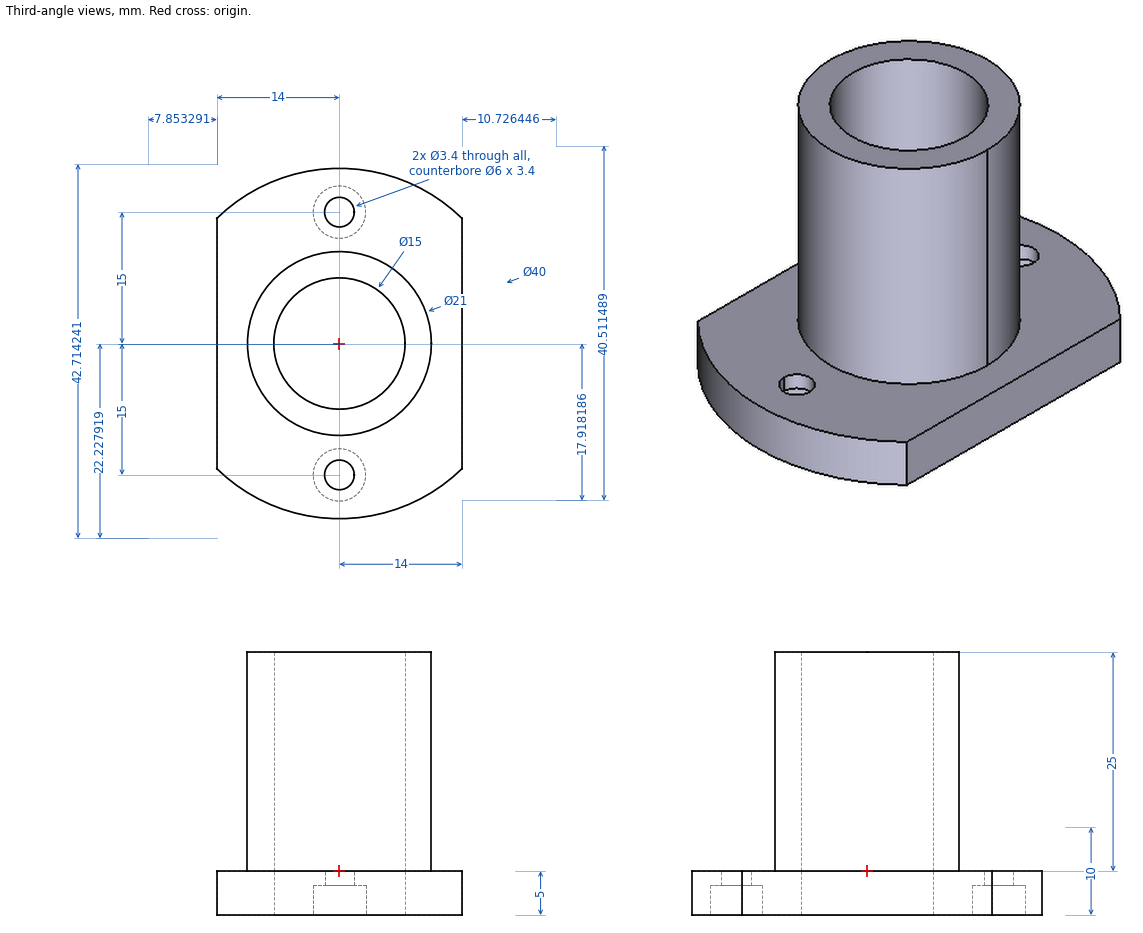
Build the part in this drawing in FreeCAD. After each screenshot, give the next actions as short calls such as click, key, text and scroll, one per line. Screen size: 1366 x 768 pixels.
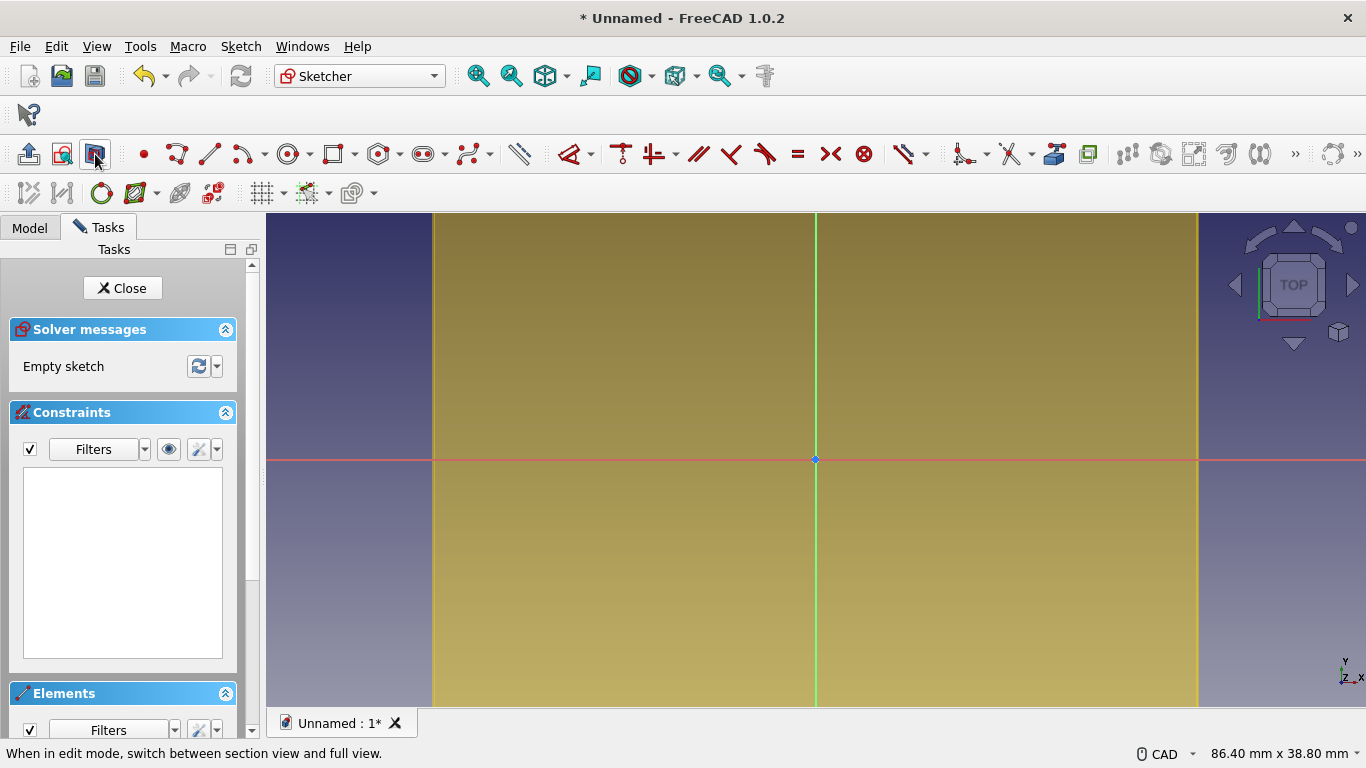
scroll(609, 460, down, 2)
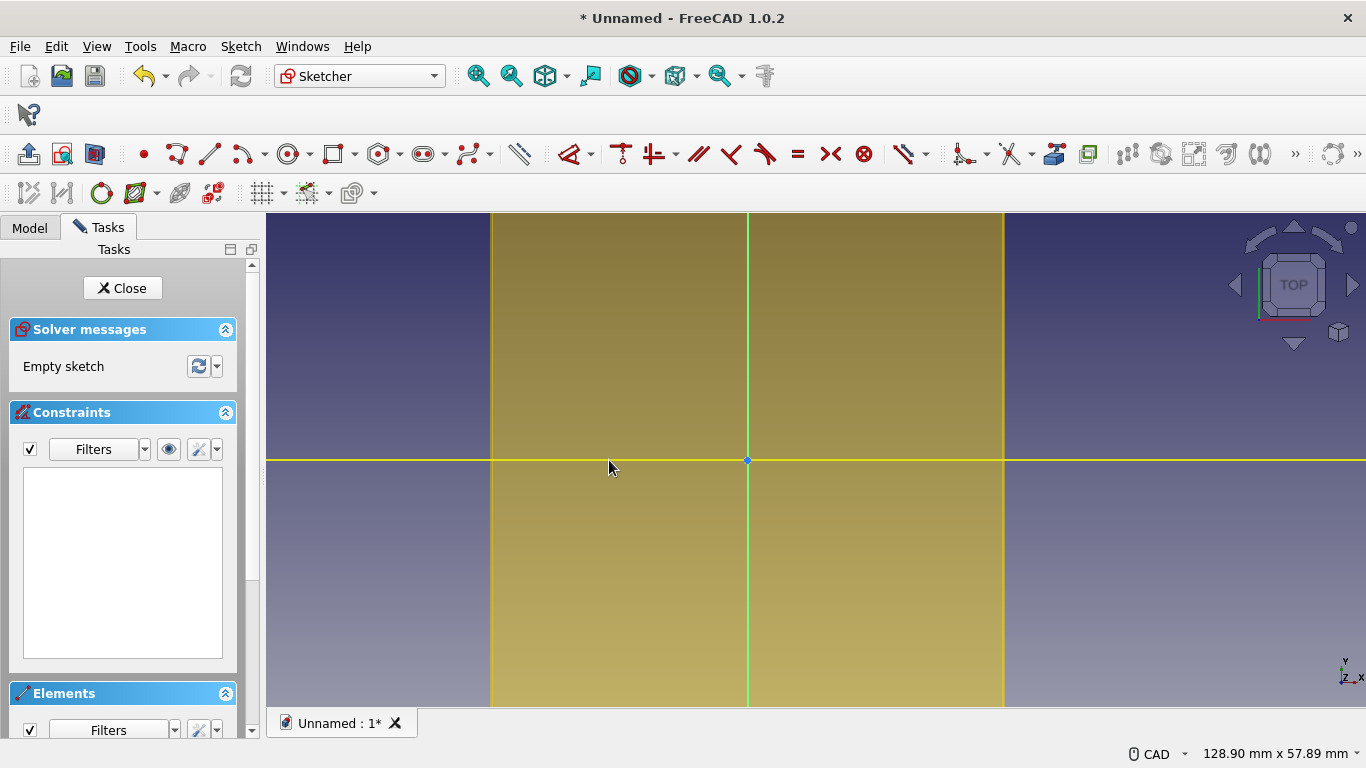
click(288, 154)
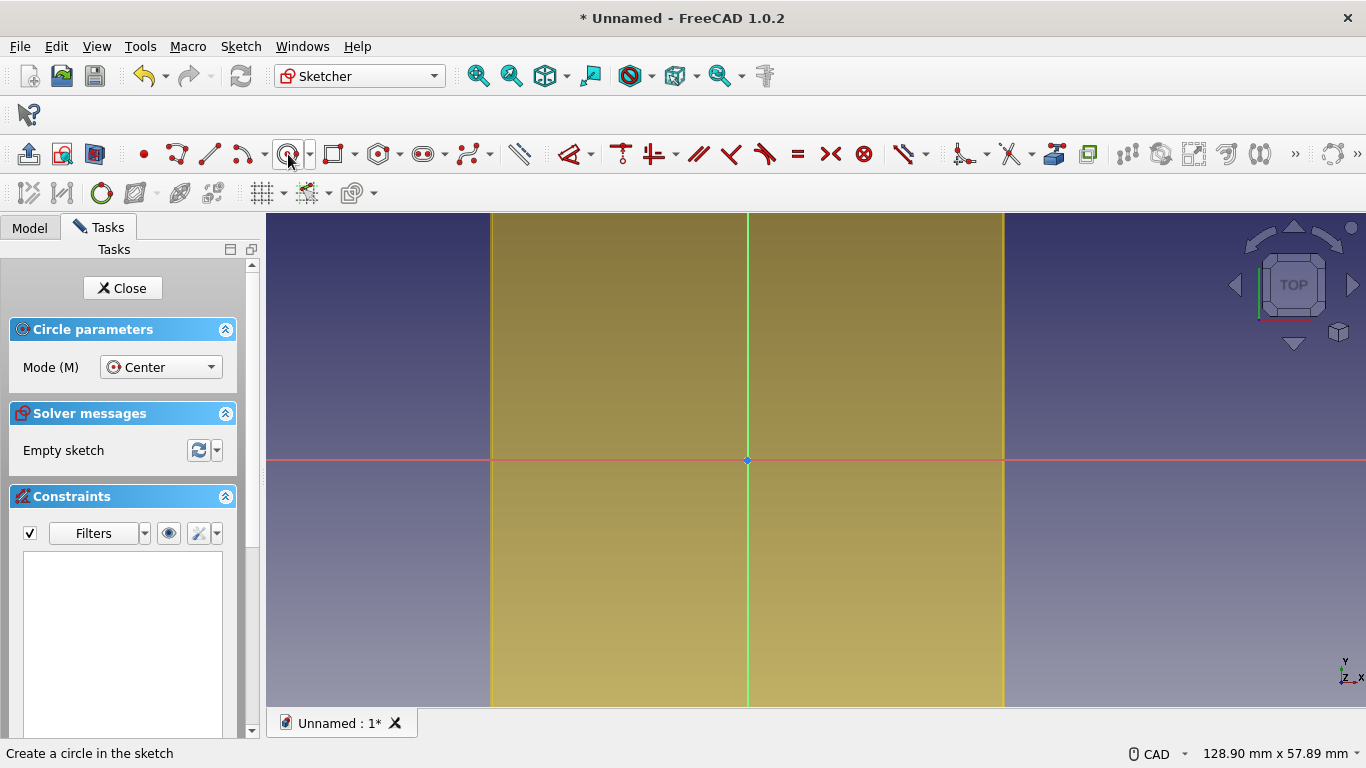
click(748, 460)
move(868, 339)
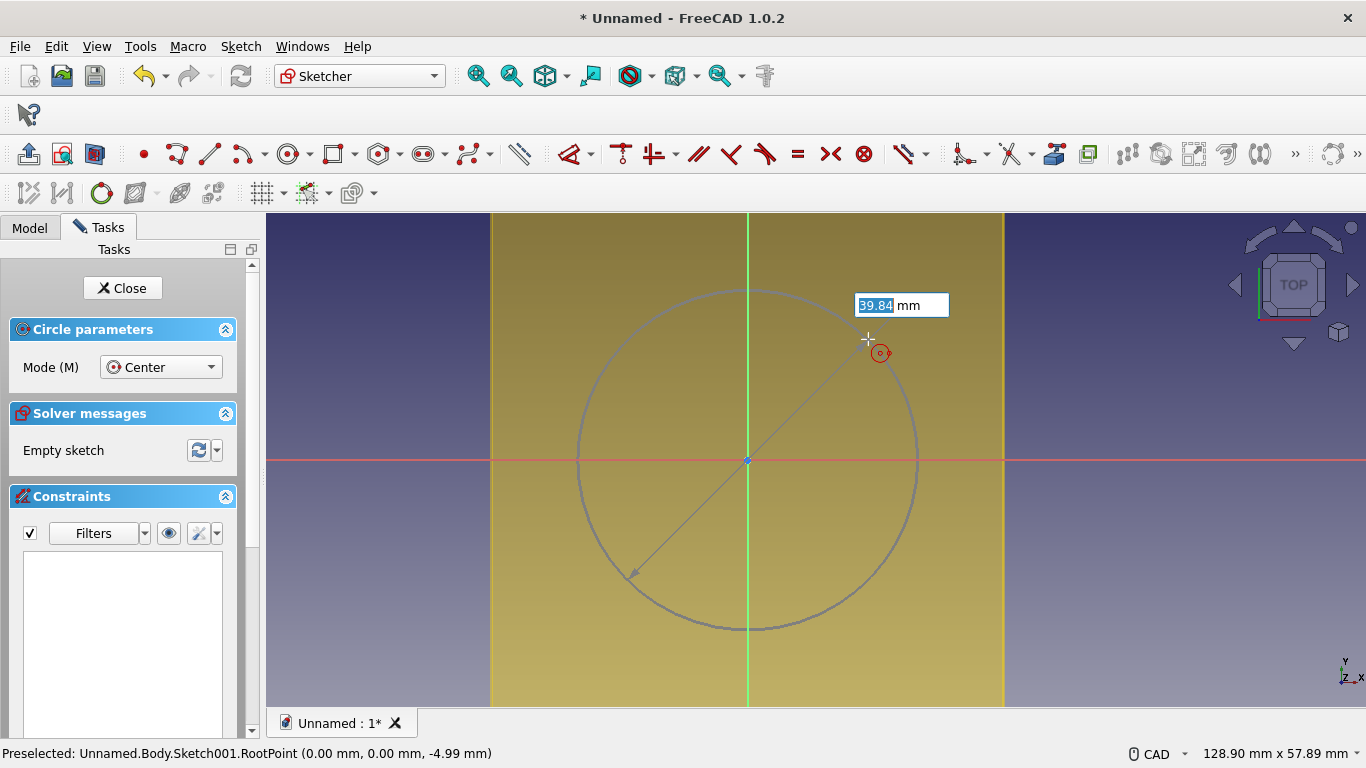
text(40)
key(Return)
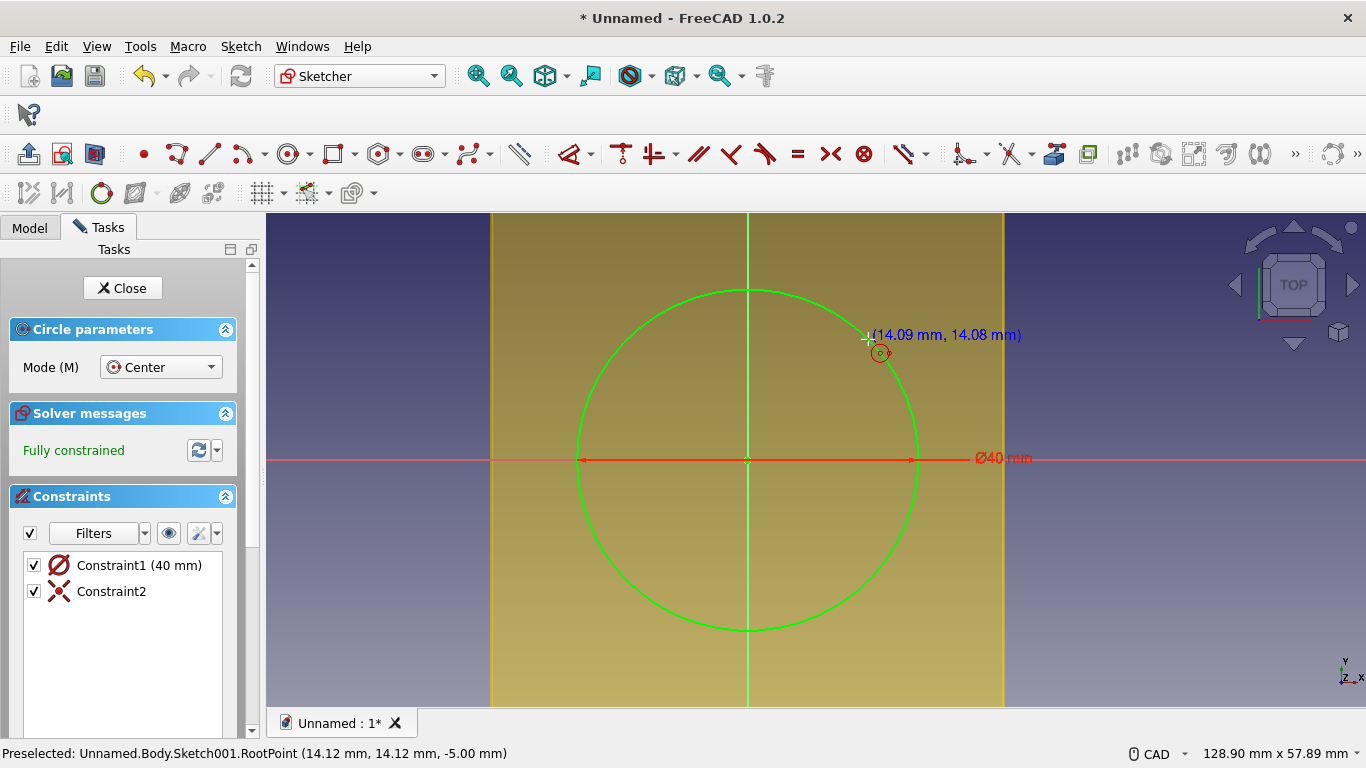
click(748, 460)
move(793, 415)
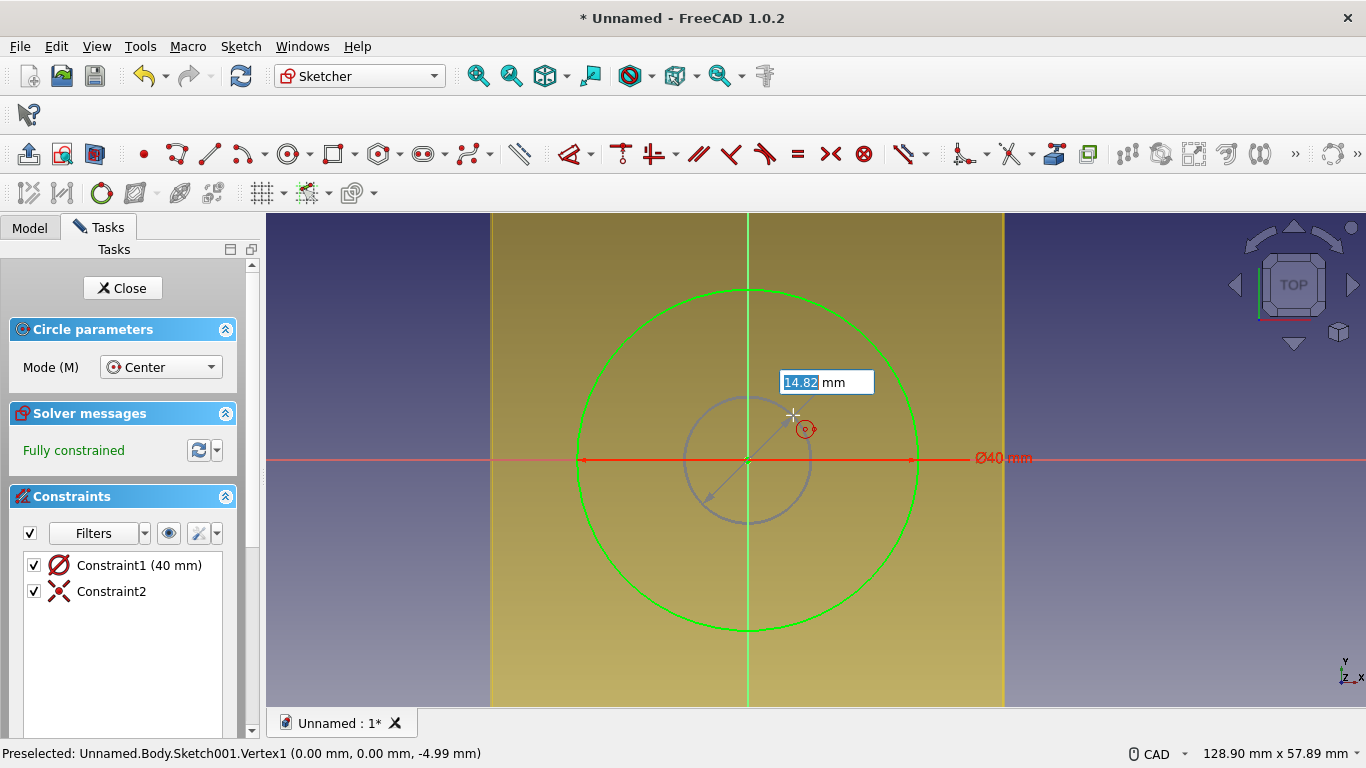
text(15)
key(Return)
key(Escape)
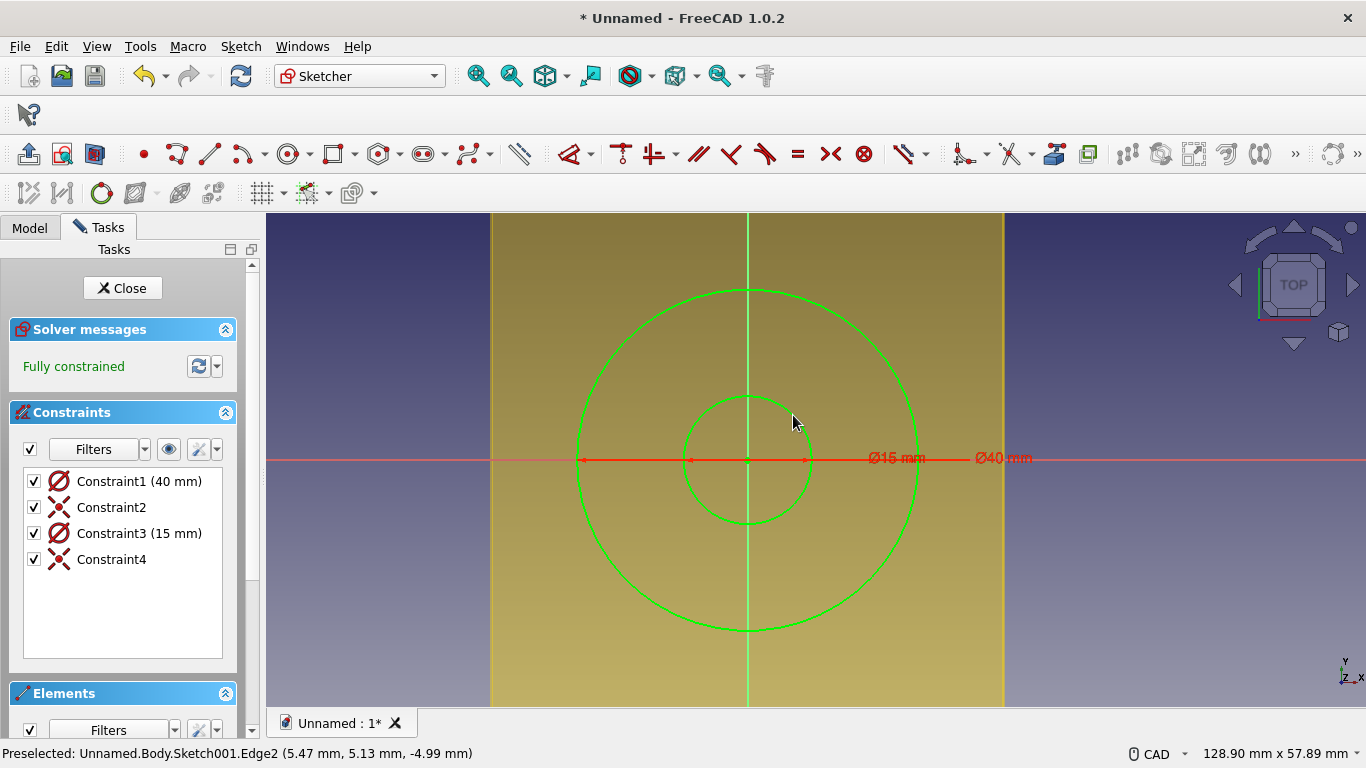
click(123, 288)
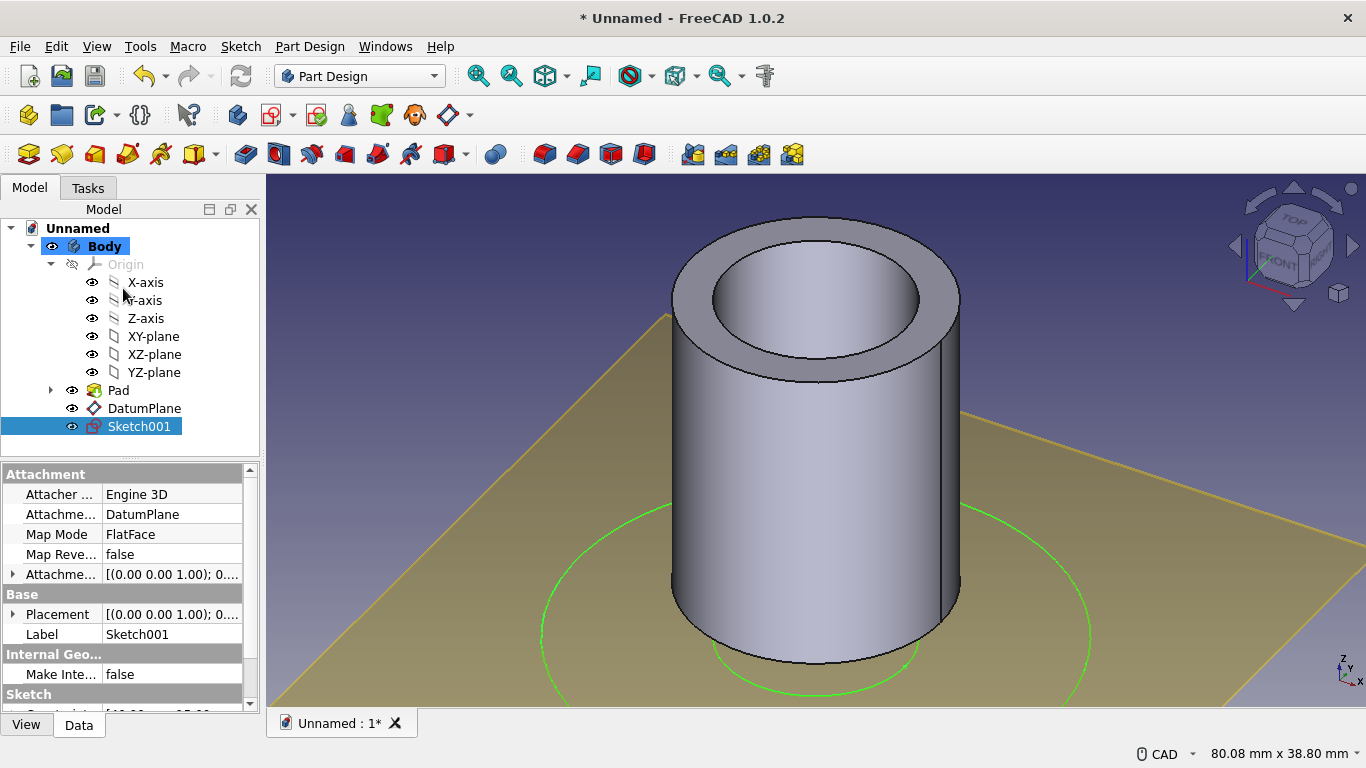
click(29, 154)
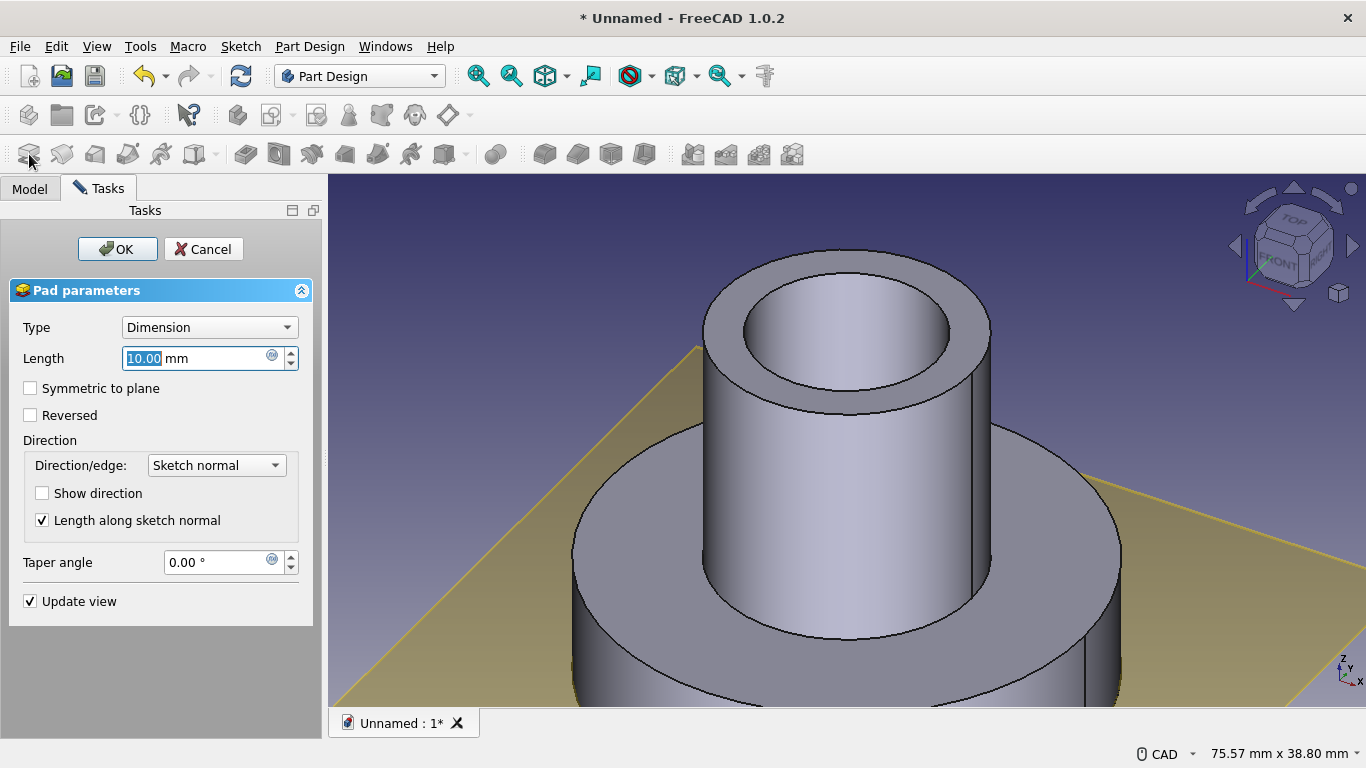
text(5)
key(Tab)